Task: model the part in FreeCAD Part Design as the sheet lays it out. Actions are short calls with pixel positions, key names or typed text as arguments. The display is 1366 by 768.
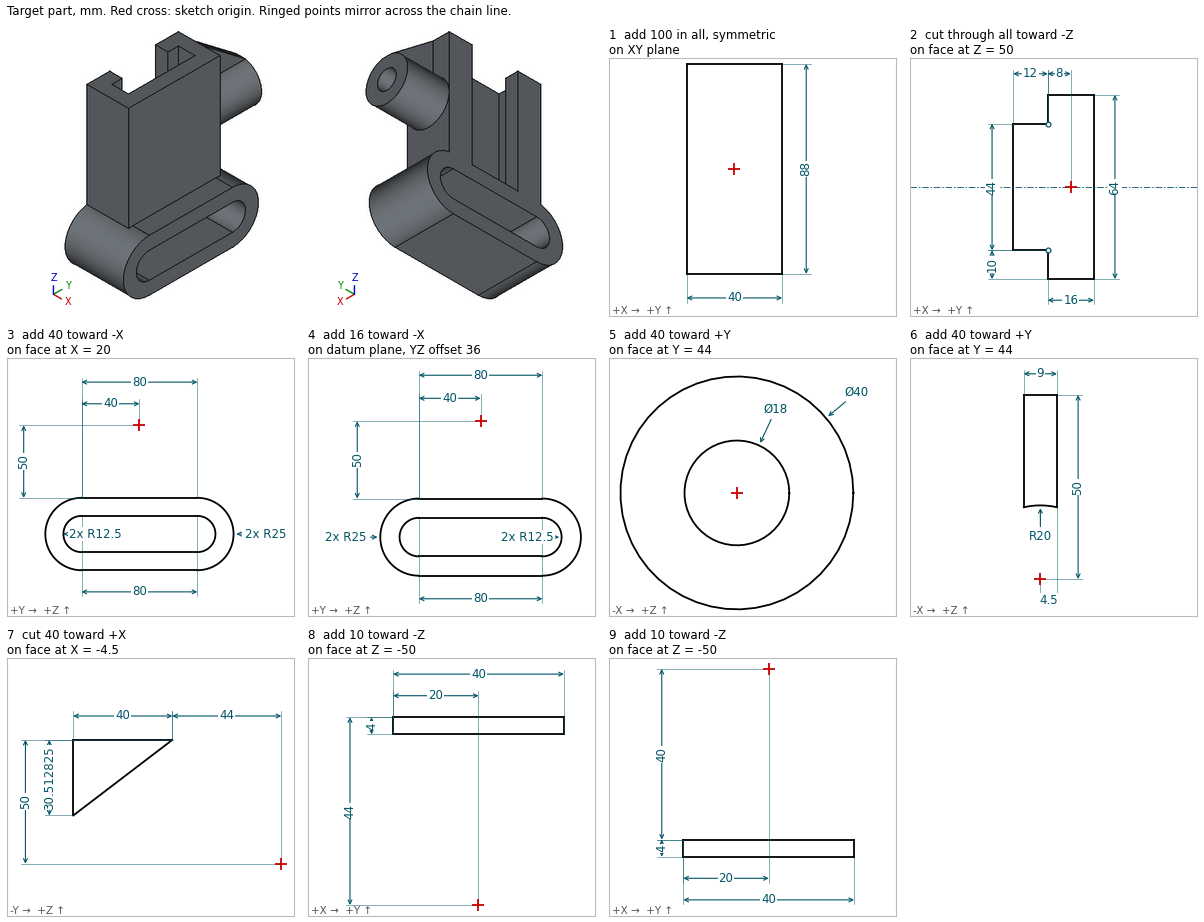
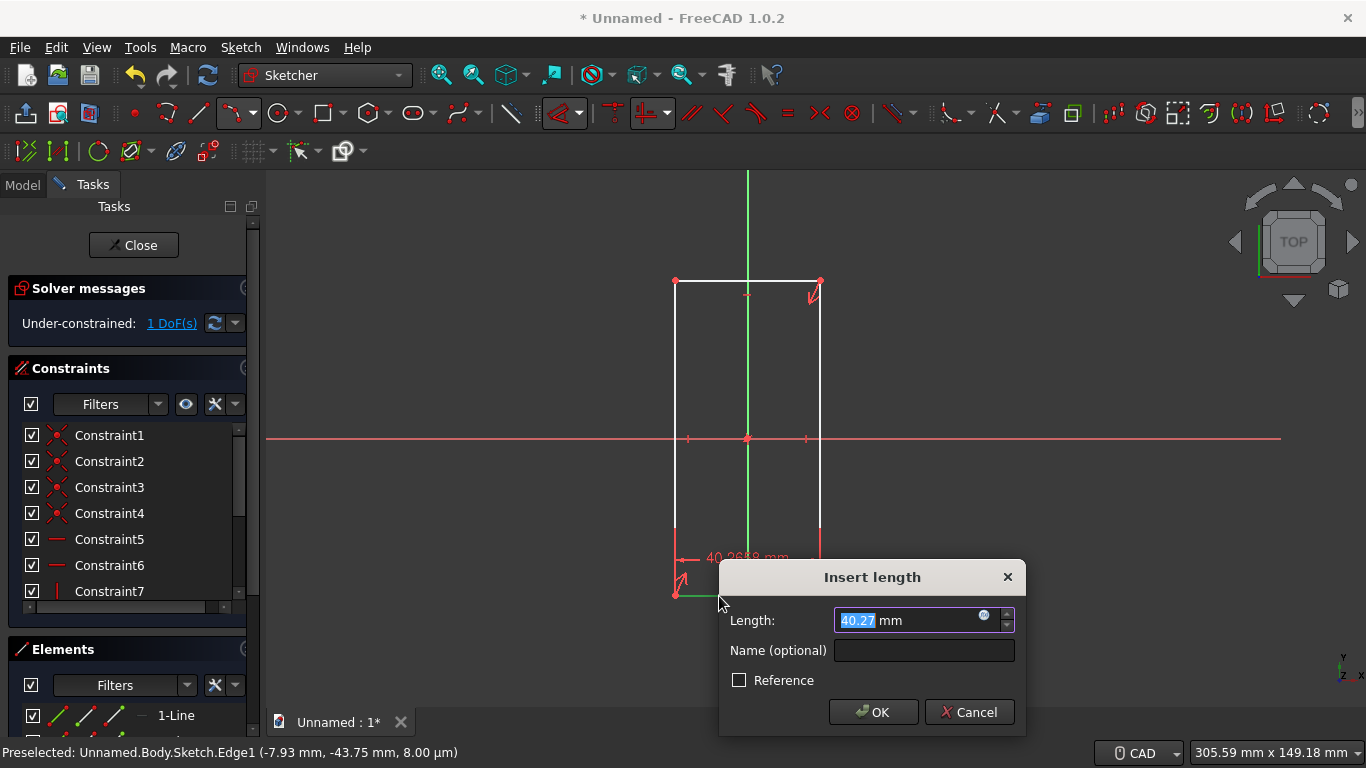
text(40)
key(Return)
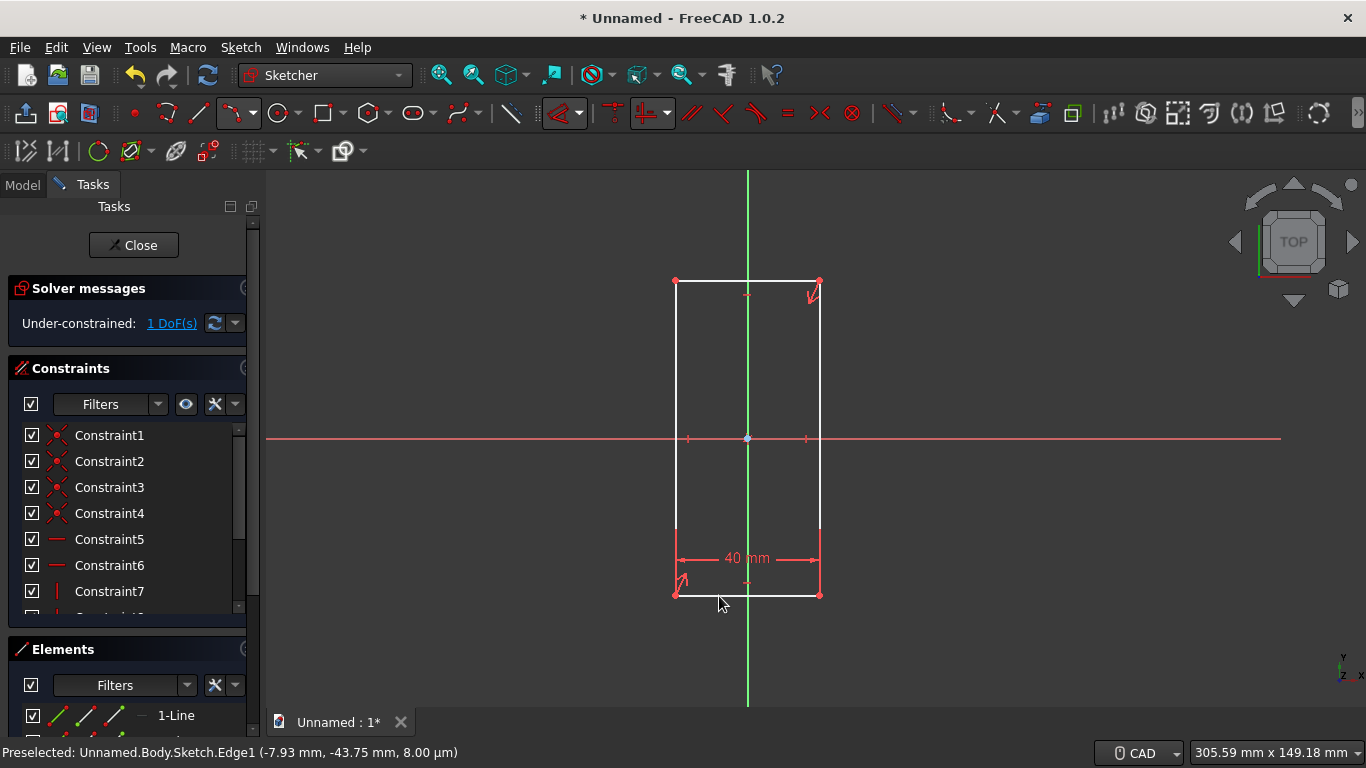
click(820, 502)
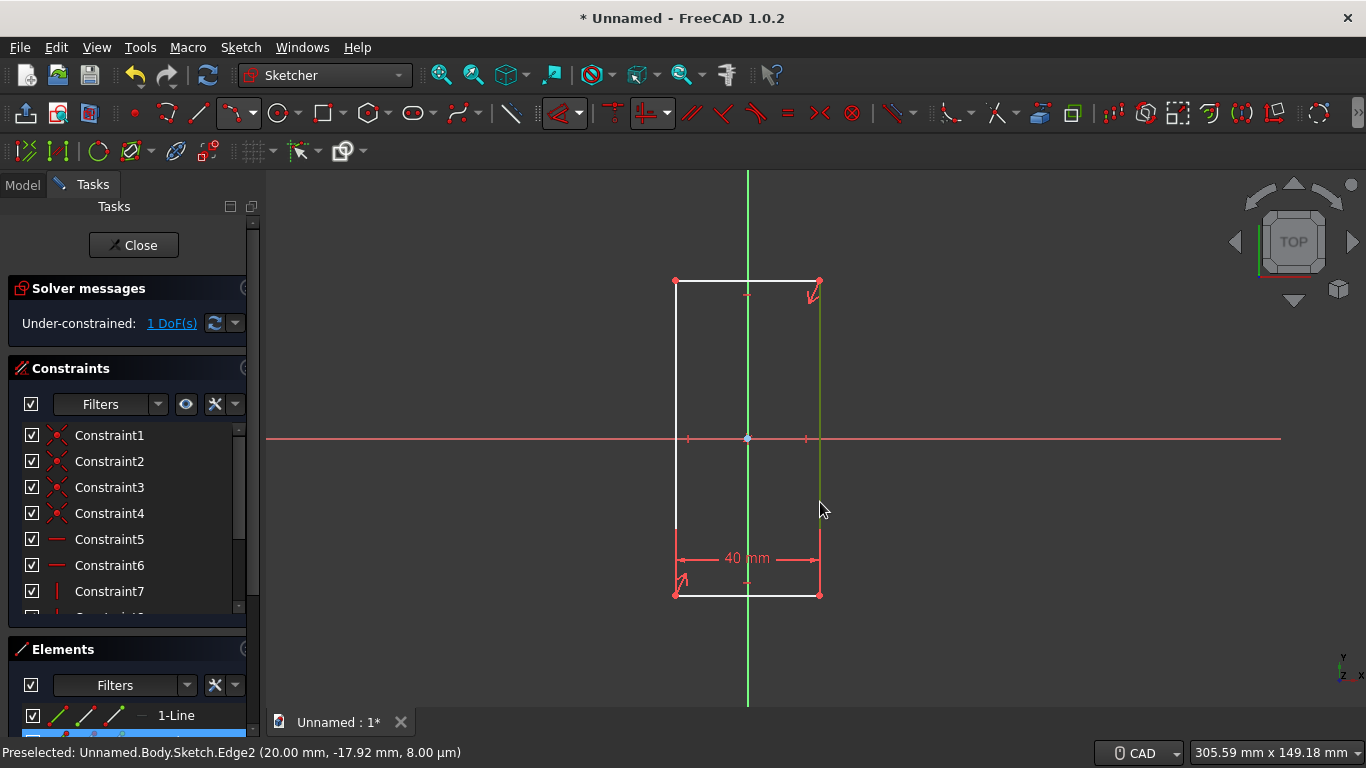
key(i)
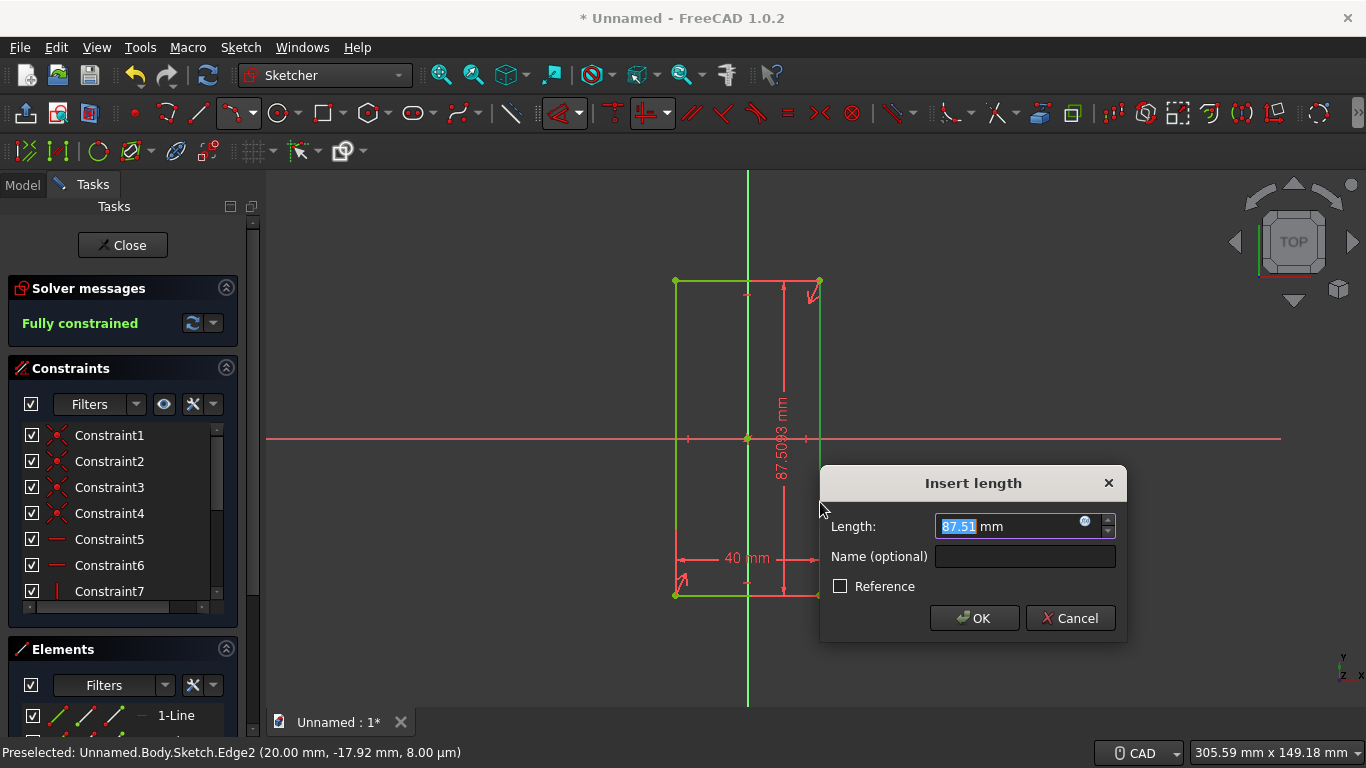
text(88)
key(Return)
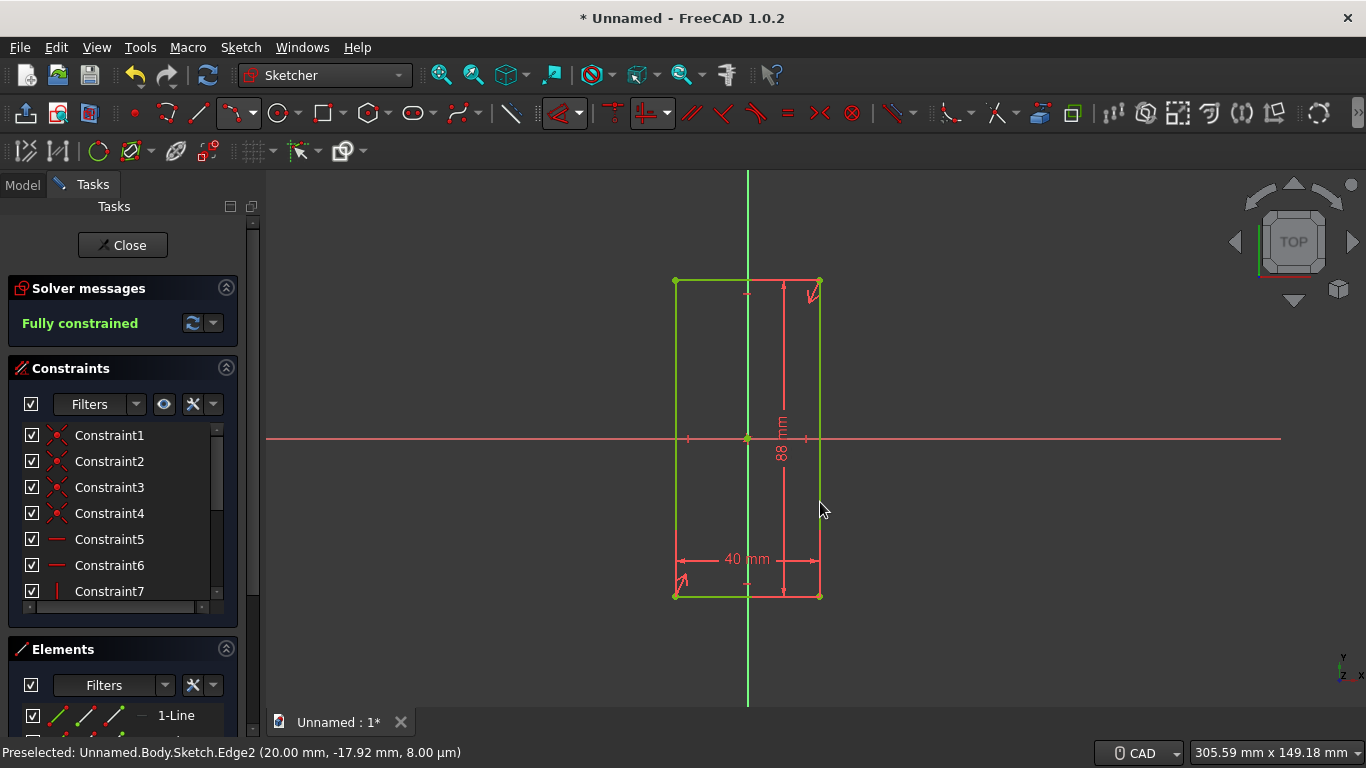
click(123, 245)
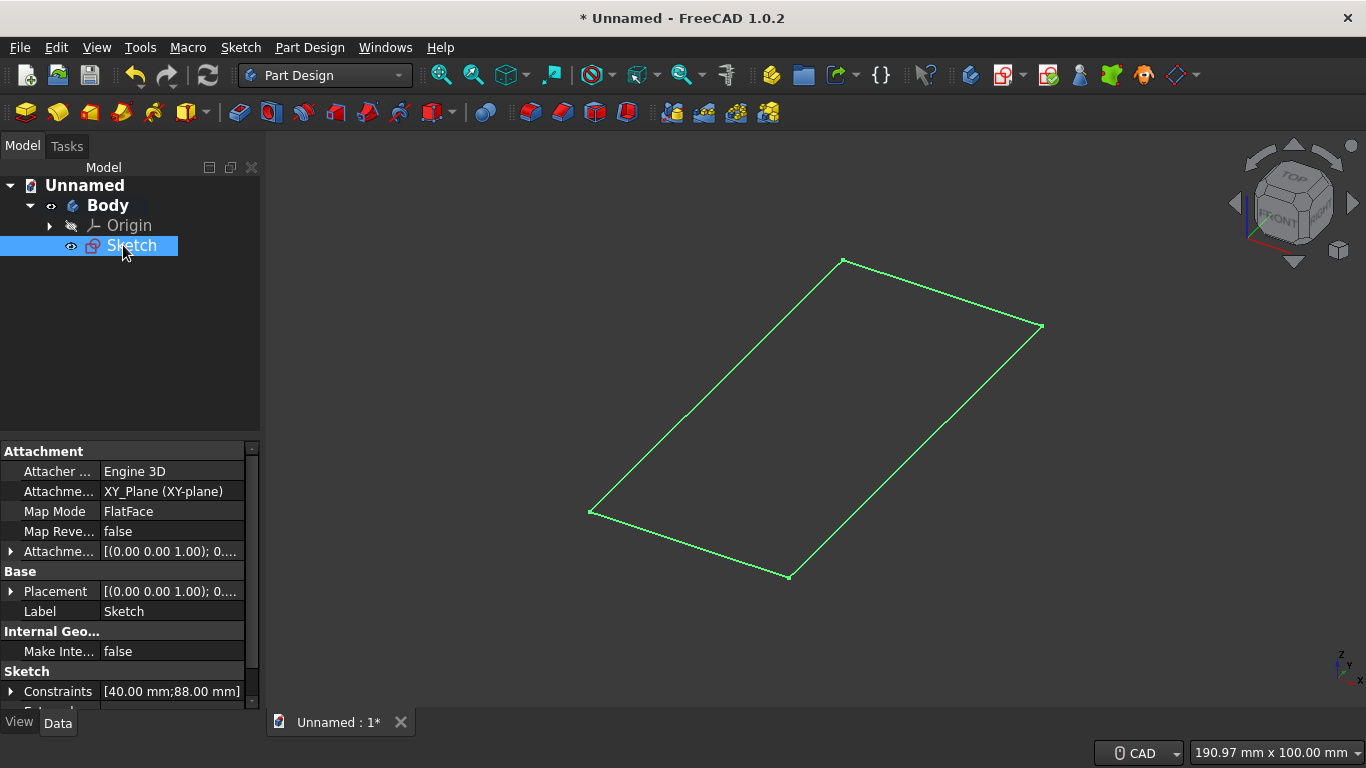
click(26, 112)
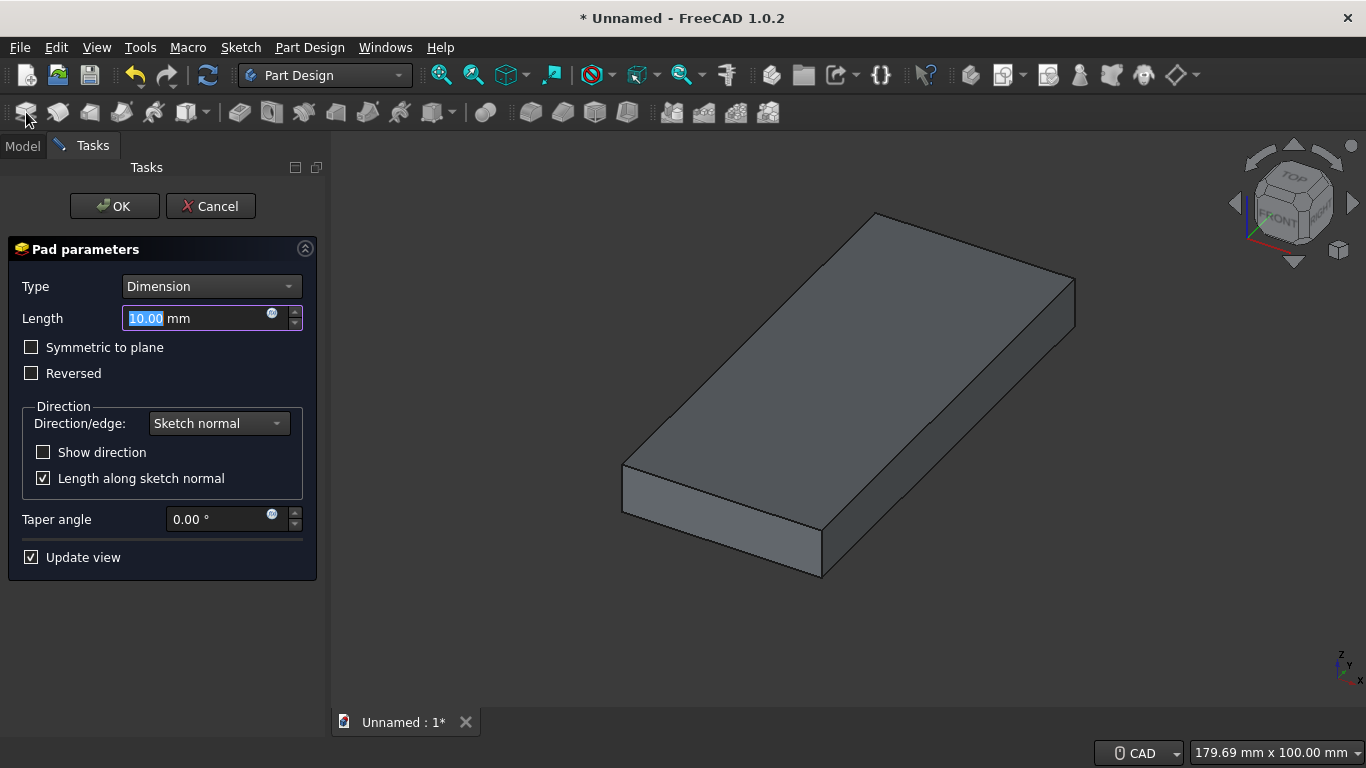
text(100)
key(Tab)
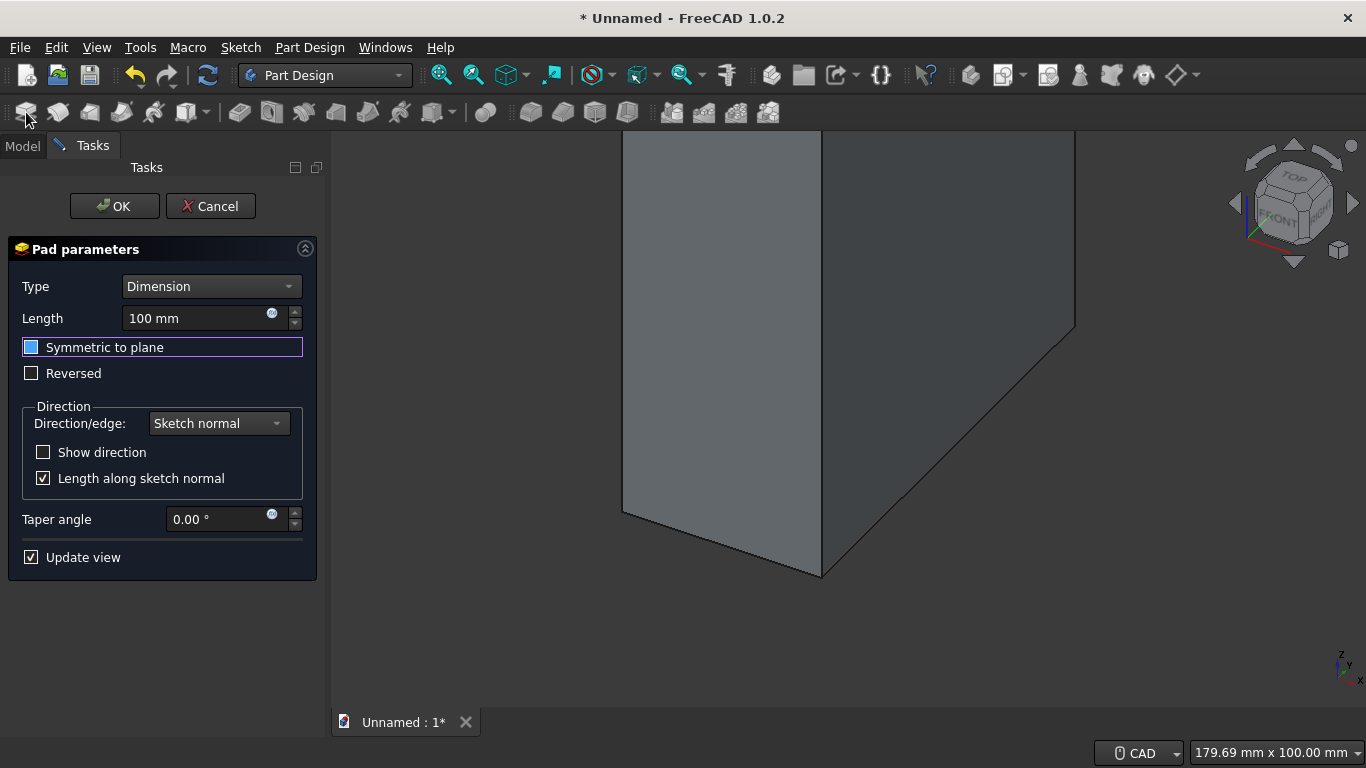
click(30, 347)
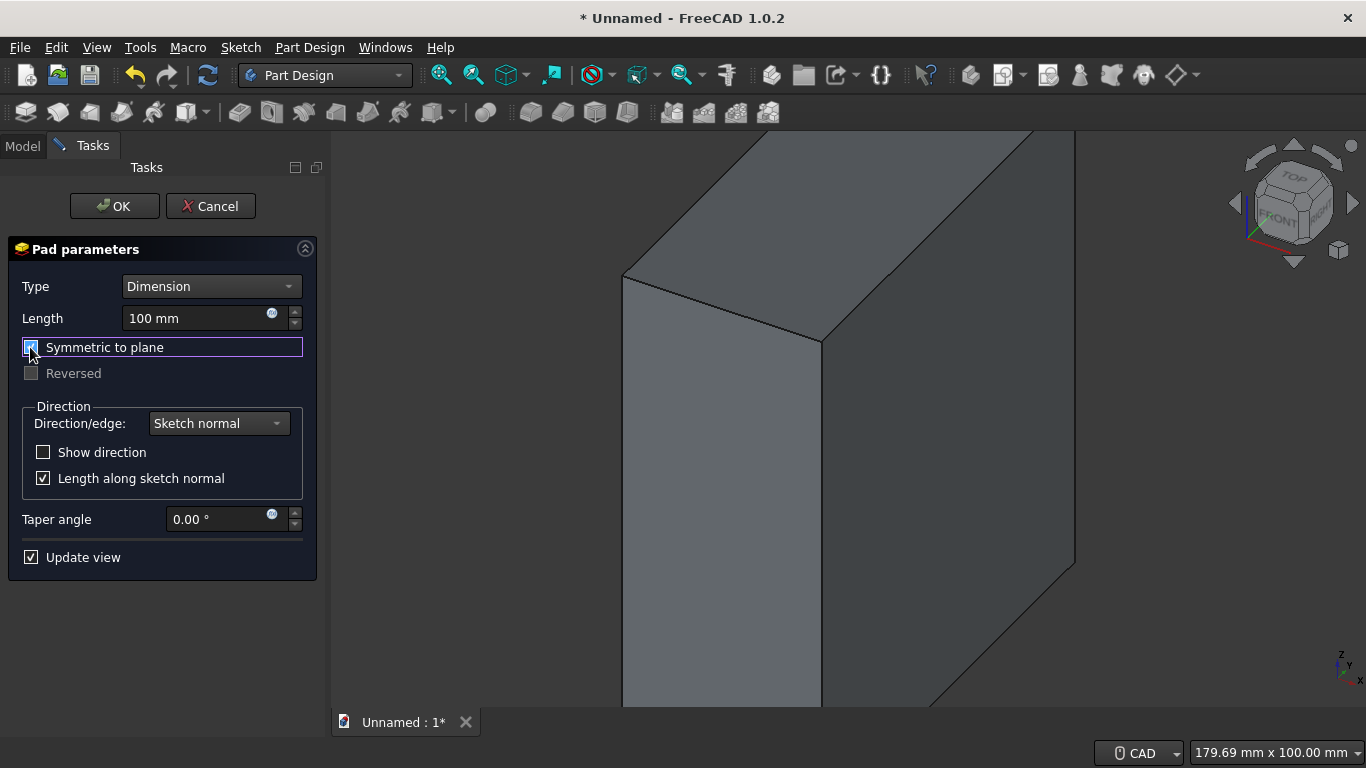
click(115, 206)